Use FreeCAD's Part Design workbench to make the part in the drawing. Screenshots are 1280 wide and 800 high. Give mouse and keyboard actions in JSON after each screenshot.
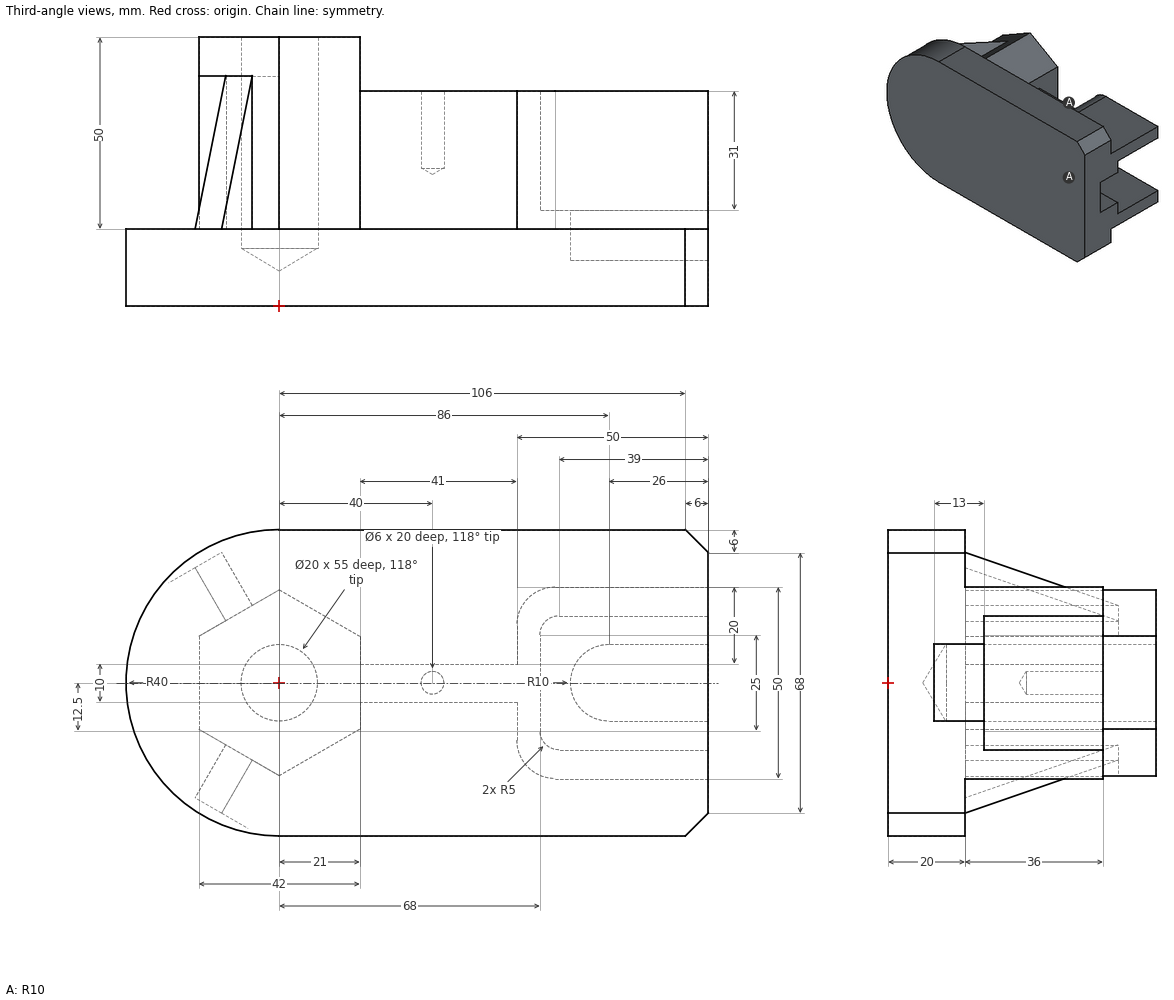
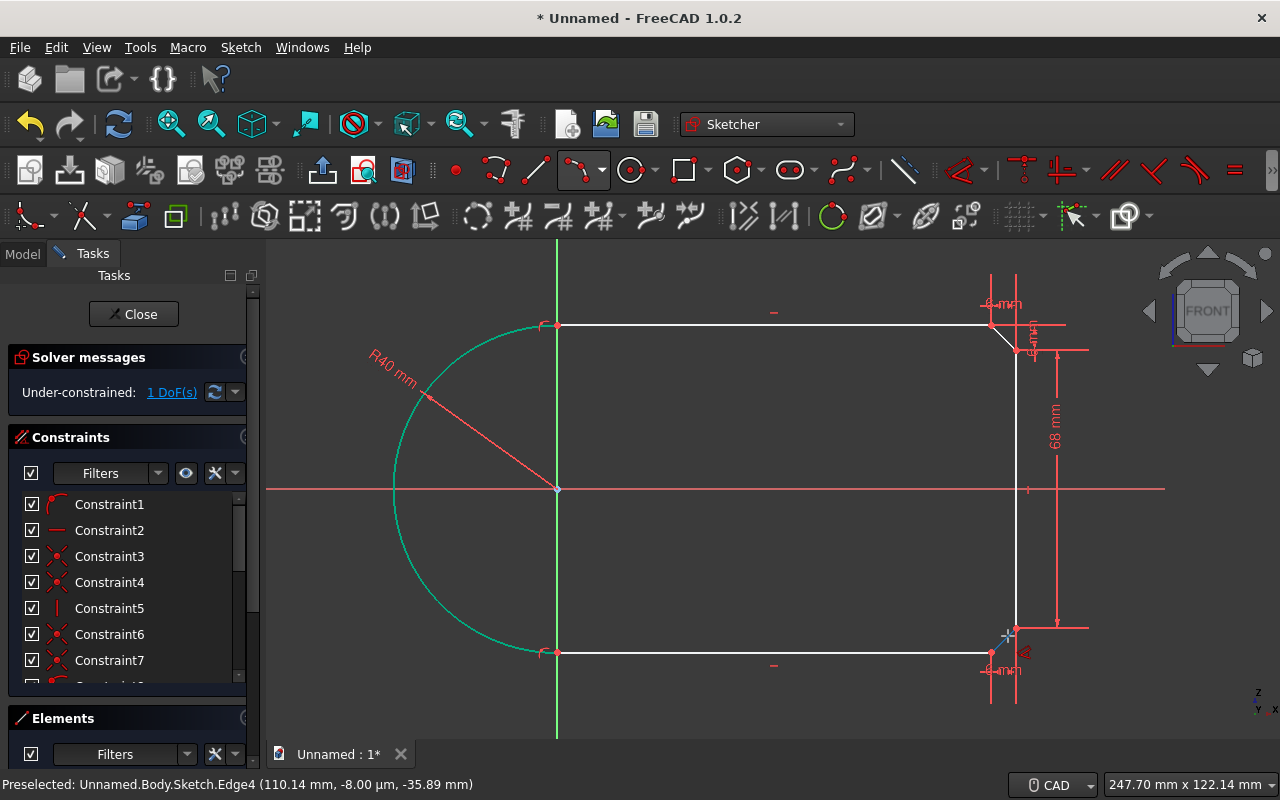
{"action": "left_click", "coordinate": [688, 325]}
{"action": "left_click", "coordinate": [774, 291]}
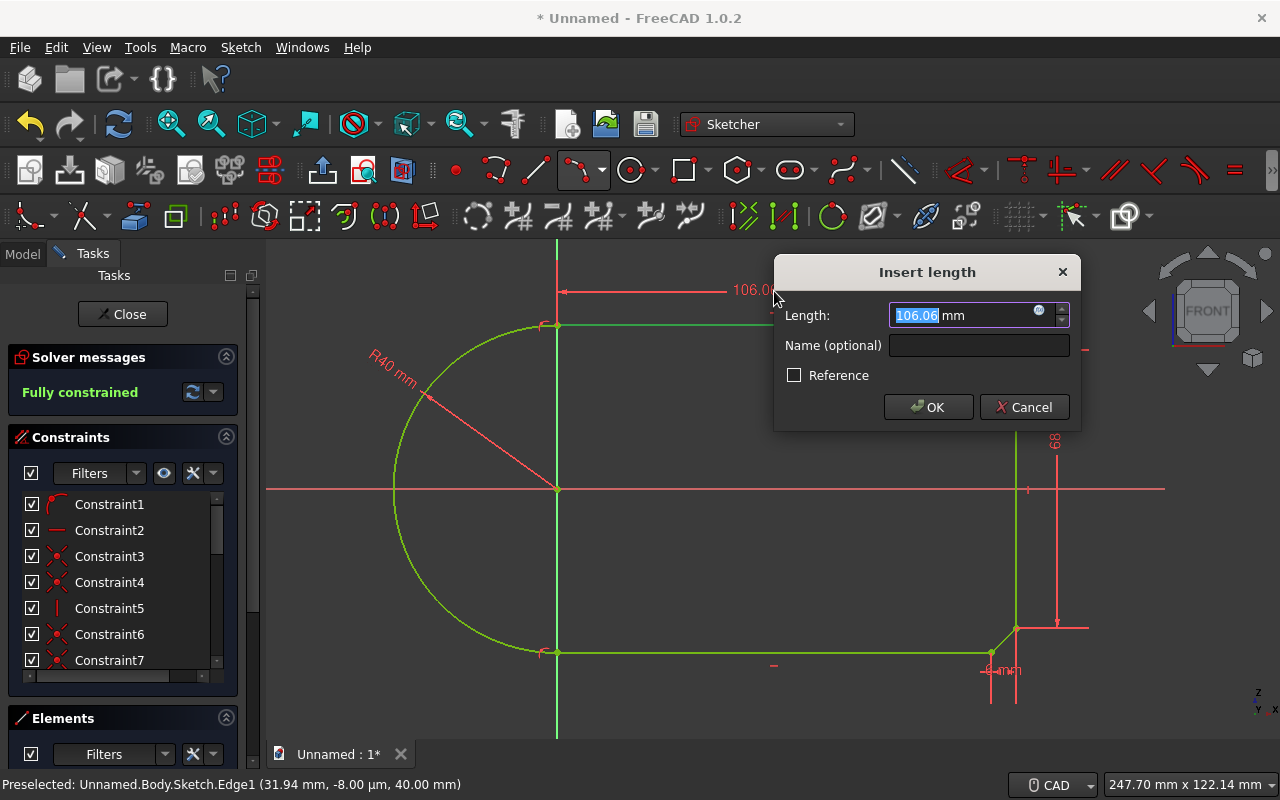
{"action": "type", "text": "106"}
{"action": "key", "text": "Return"}
{"action": "key", "text": "Escape"}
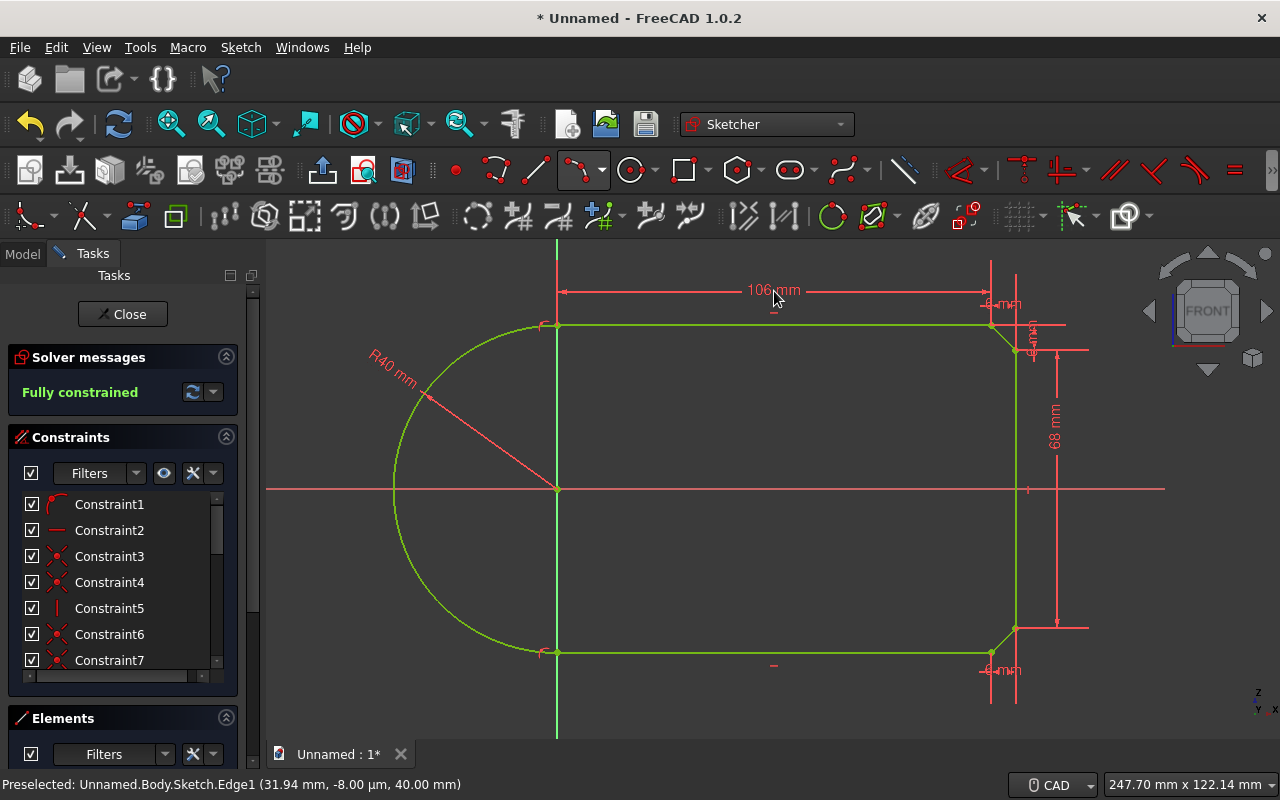
{"action": "left_click", "coordinate": [123, 314]}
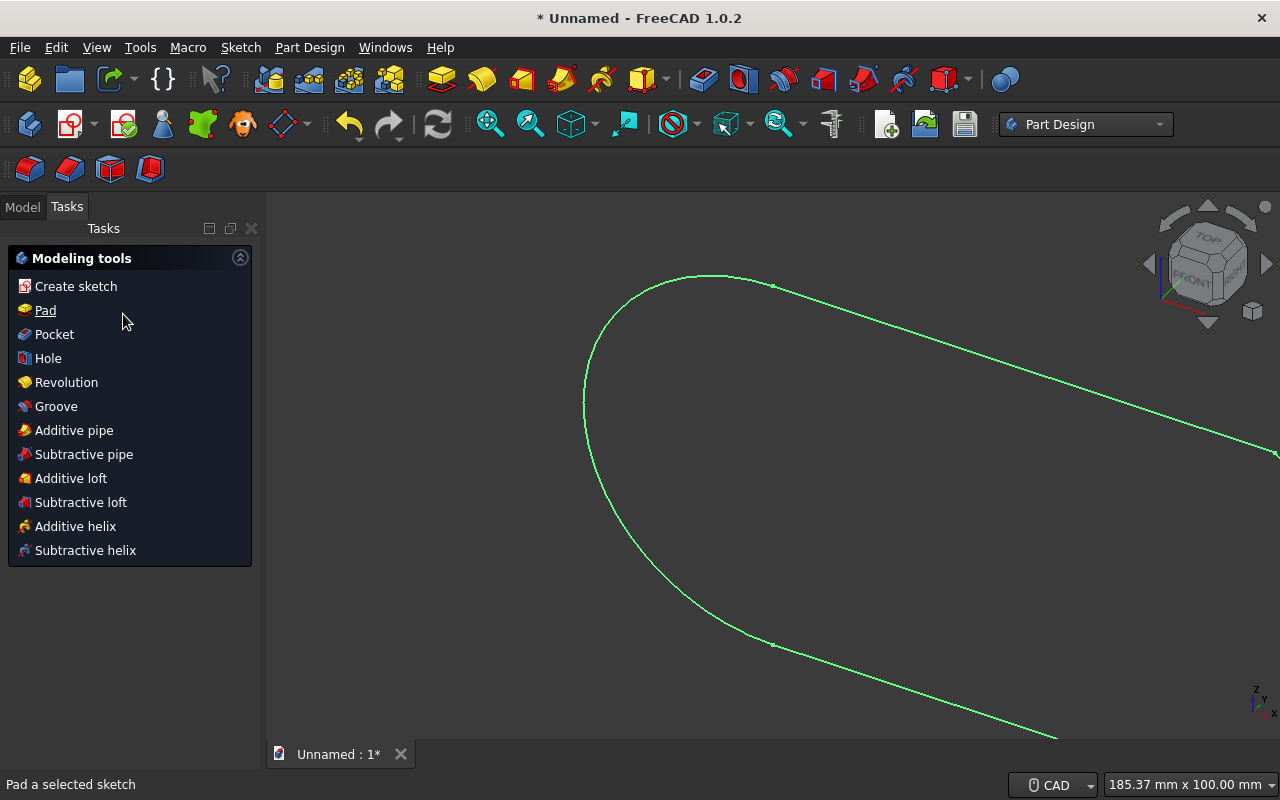
{"action": "left_click", "coordinate": [442, 80]}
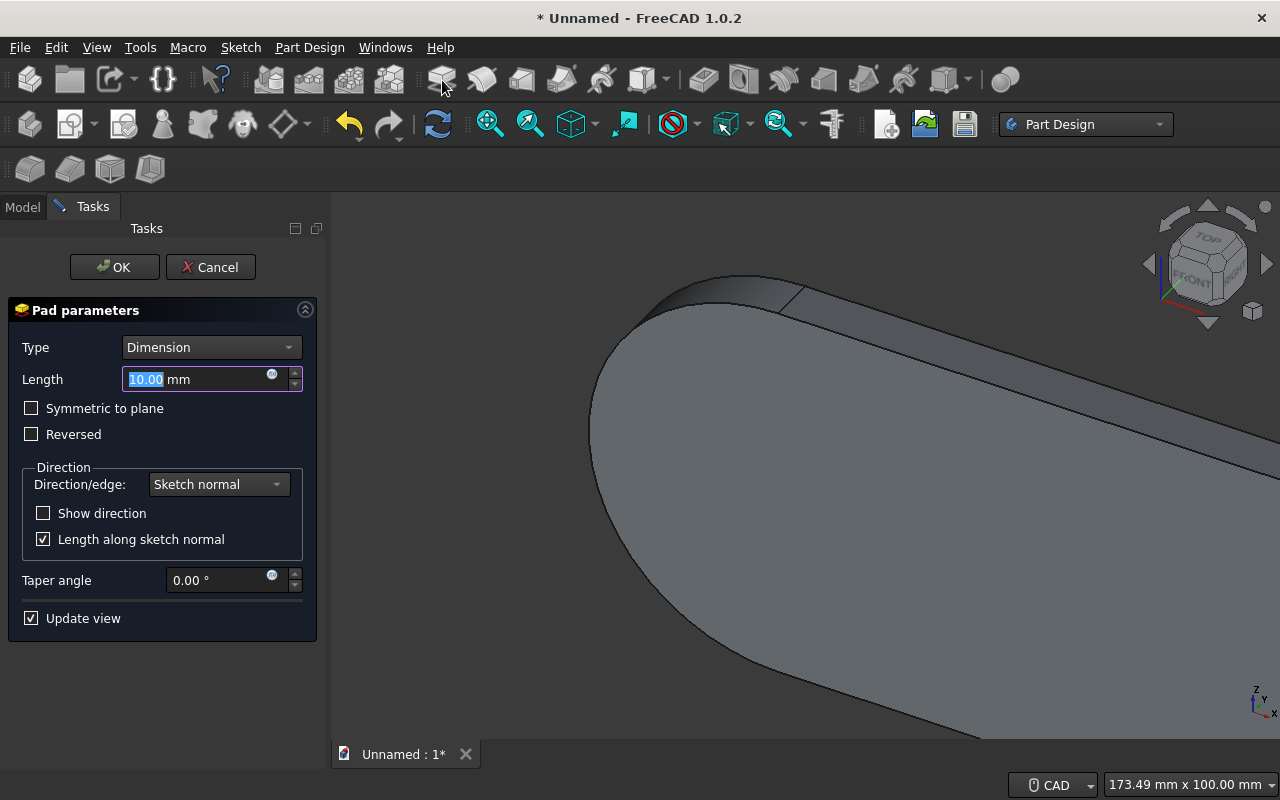
{"action": "type", "text": "20"}
{"action": "key", "text": "Tab"}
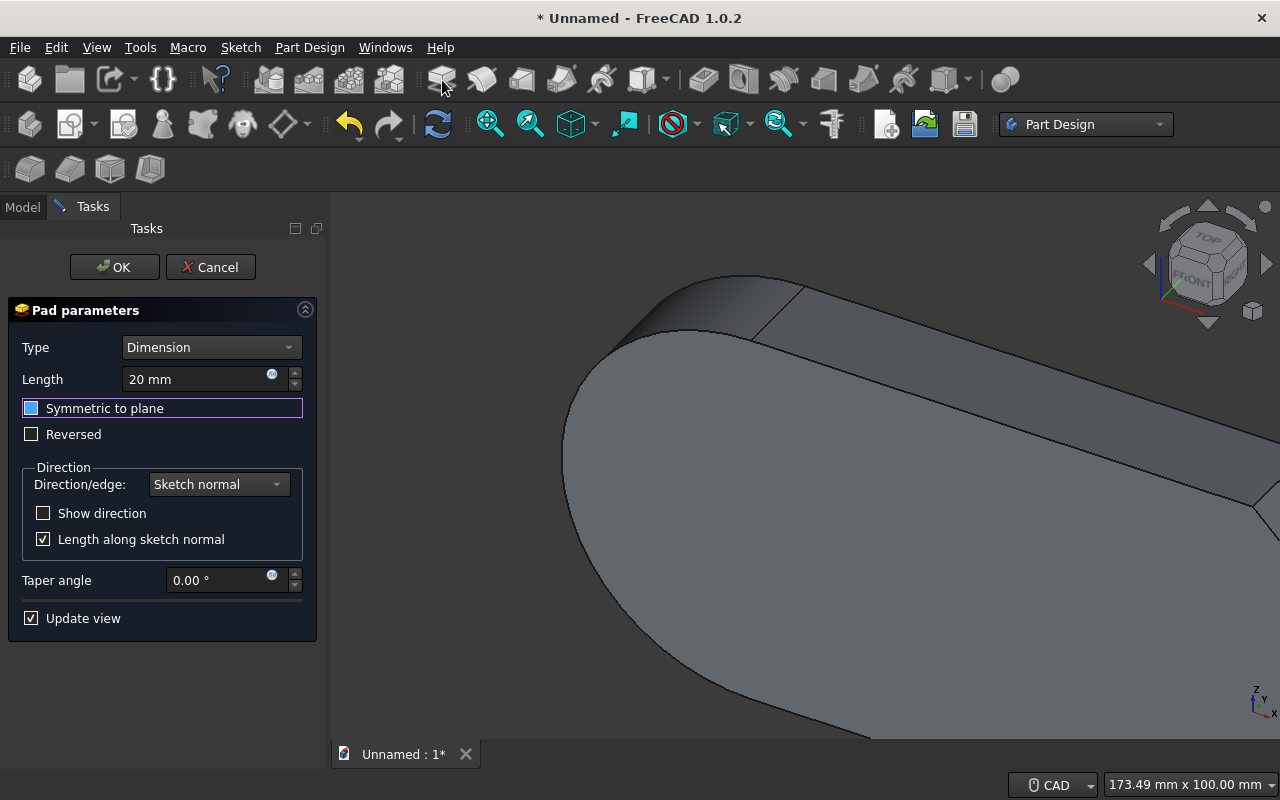
{"action": "left_click", "coordinate": [30, 434]}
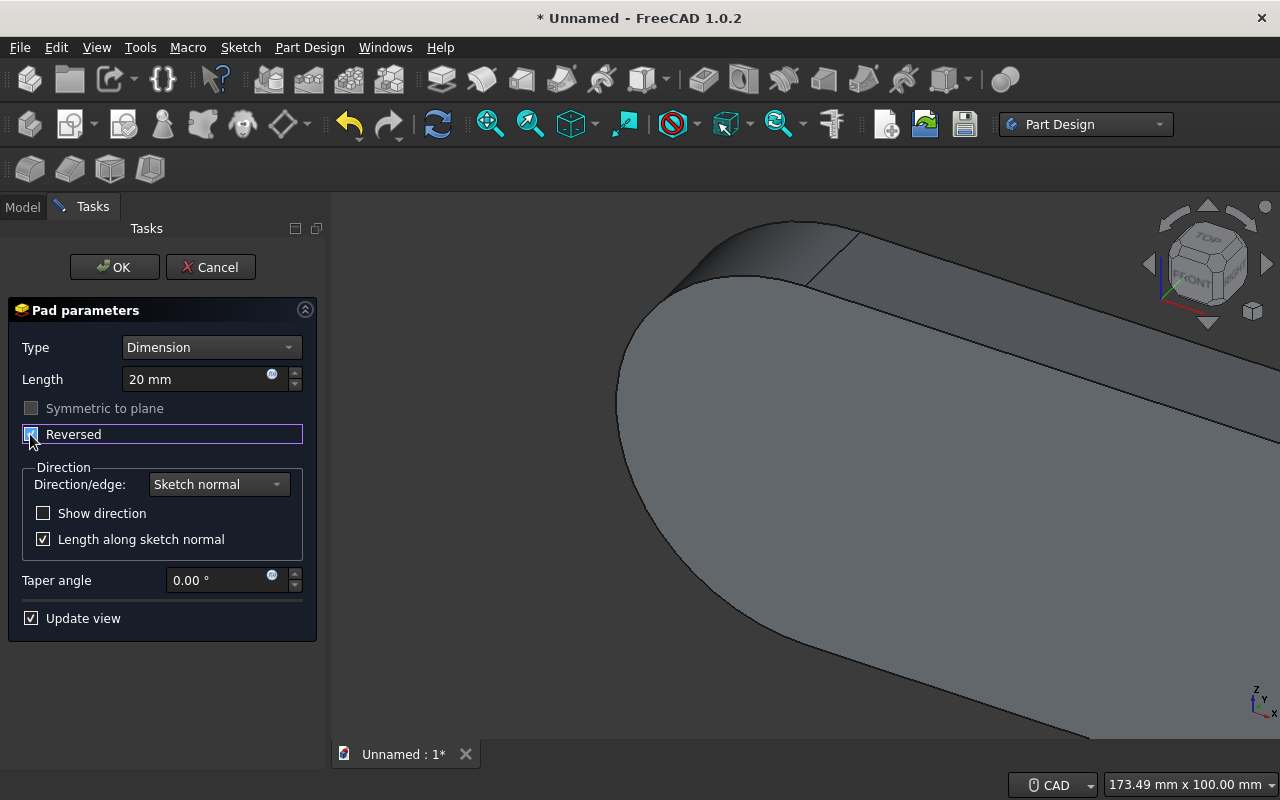
{"action": "left_click", "coordinate": [115, 267]}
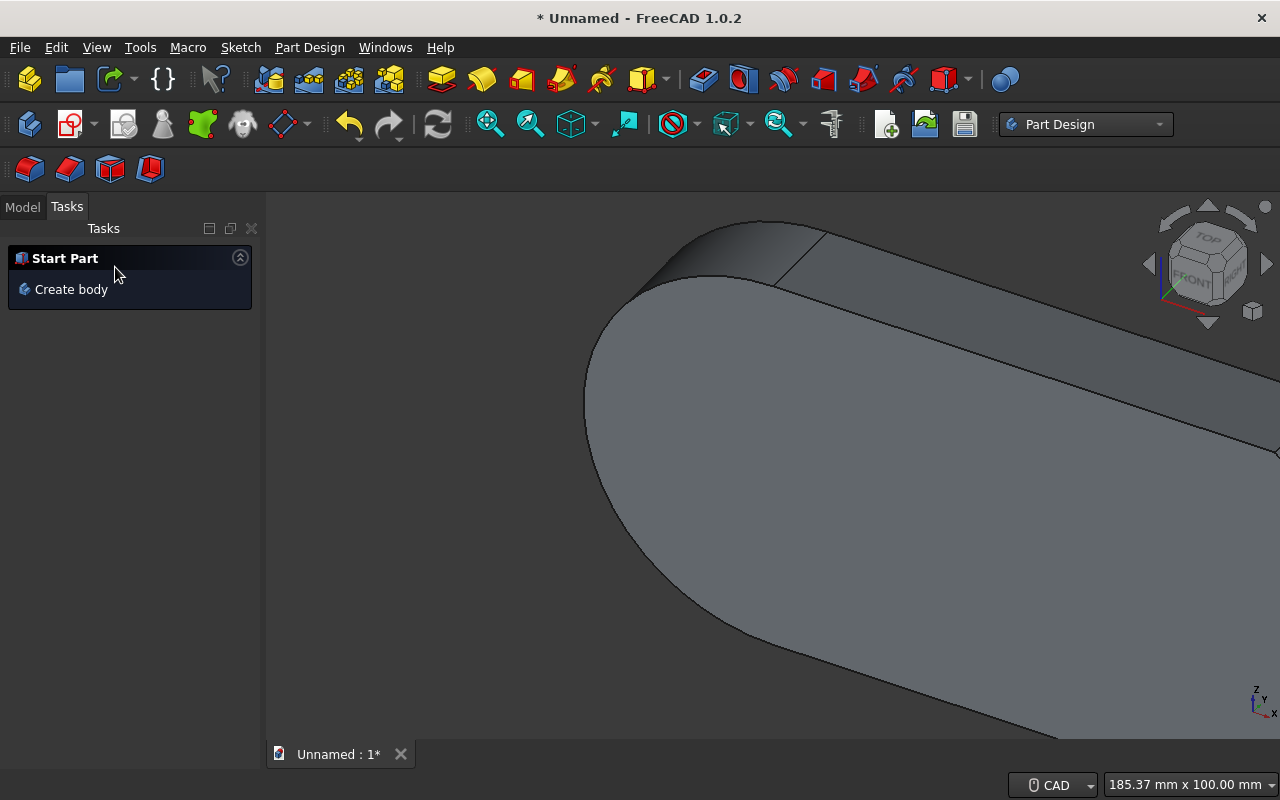
{"action": "left_click", "coordinate": [492, 124]}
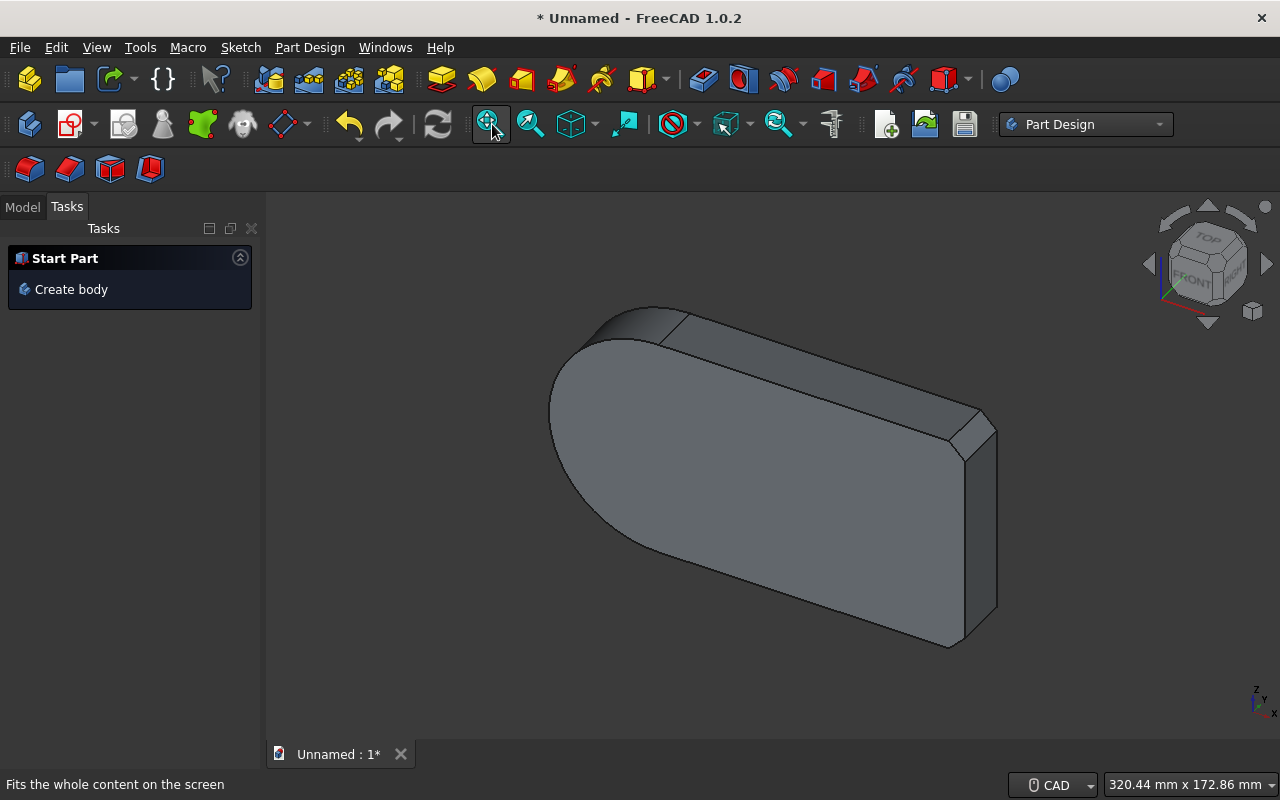
{"action": "key", "text": "4"}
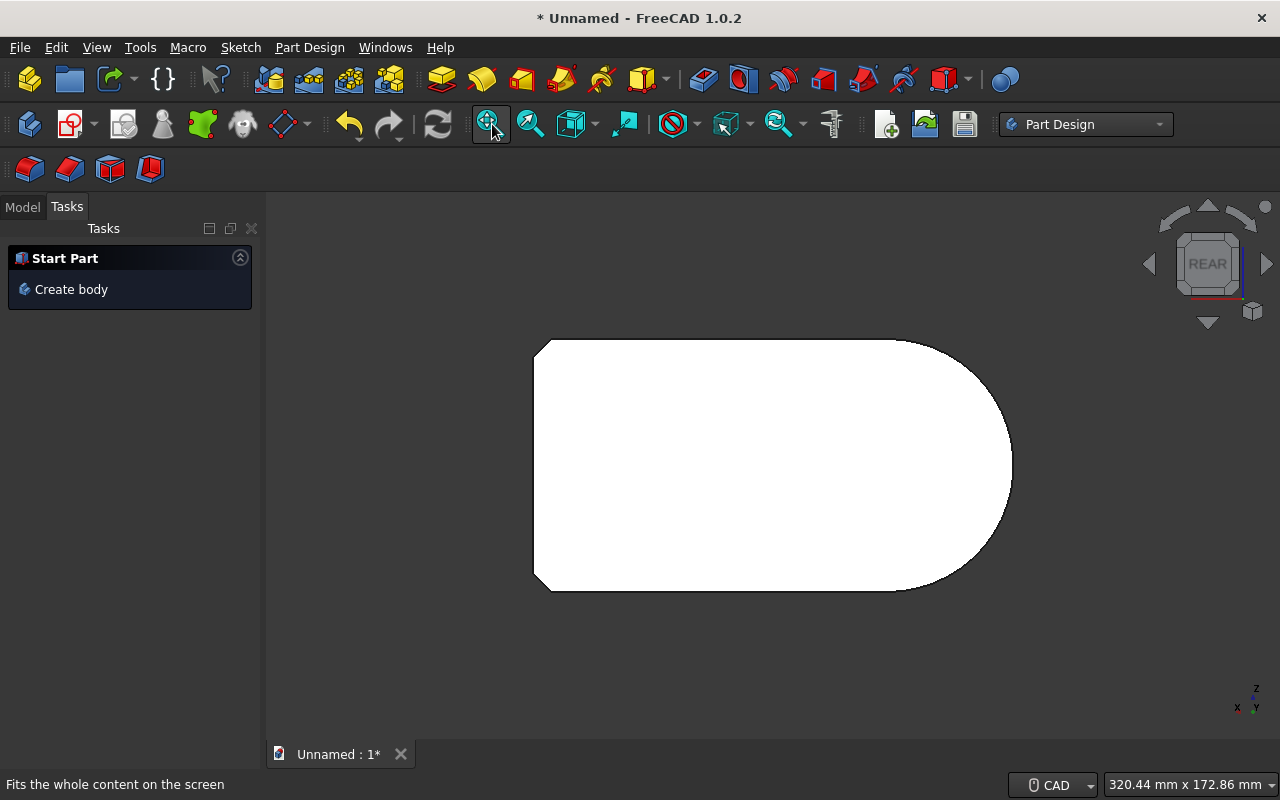
{"action": "left_click", "coordinate": [704, 465]}